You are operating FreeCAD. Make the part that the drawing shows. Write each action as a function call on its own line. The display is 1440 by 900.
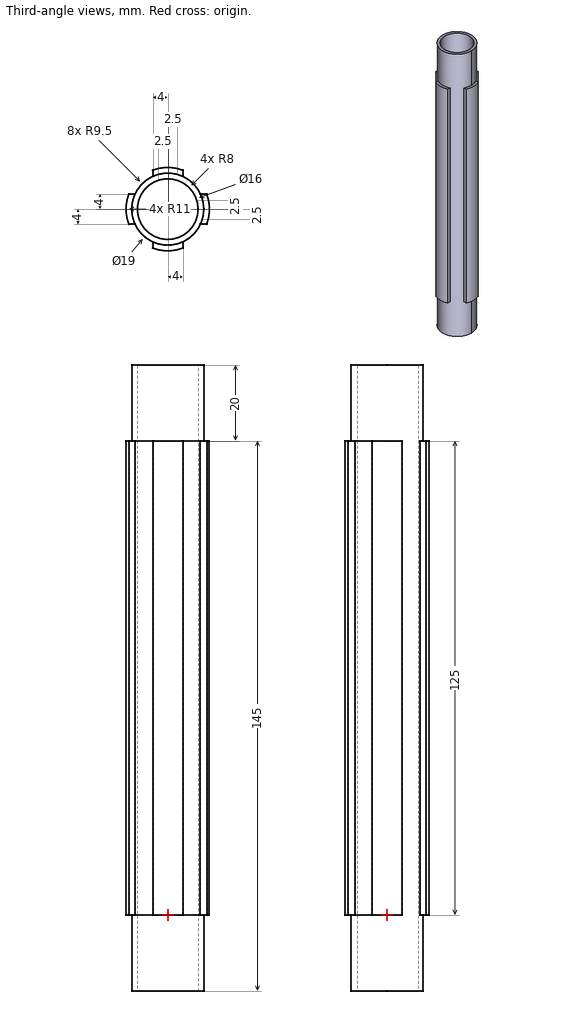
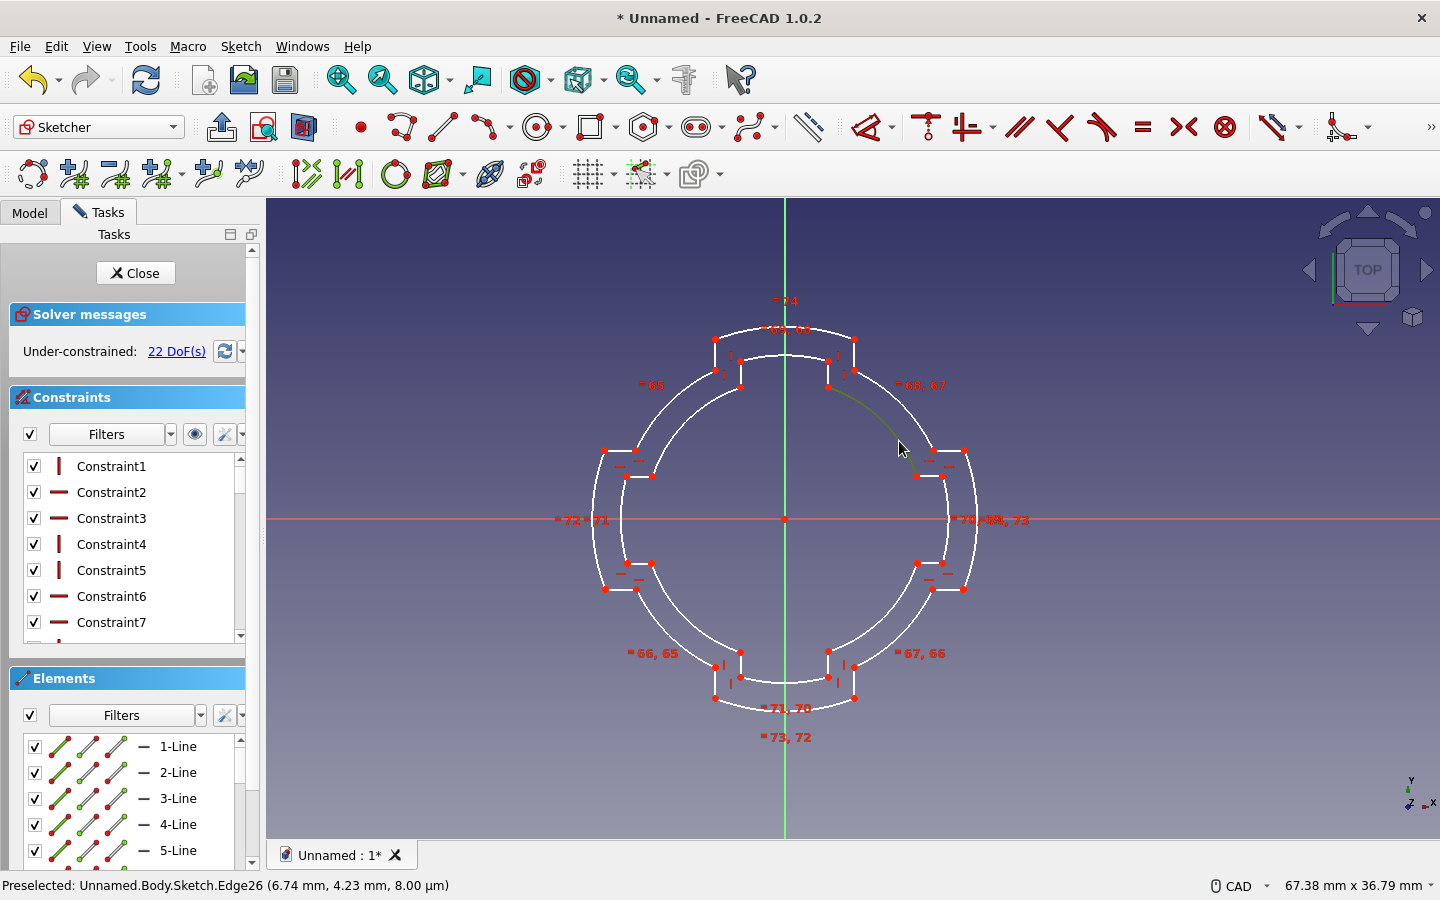
click(863, 635)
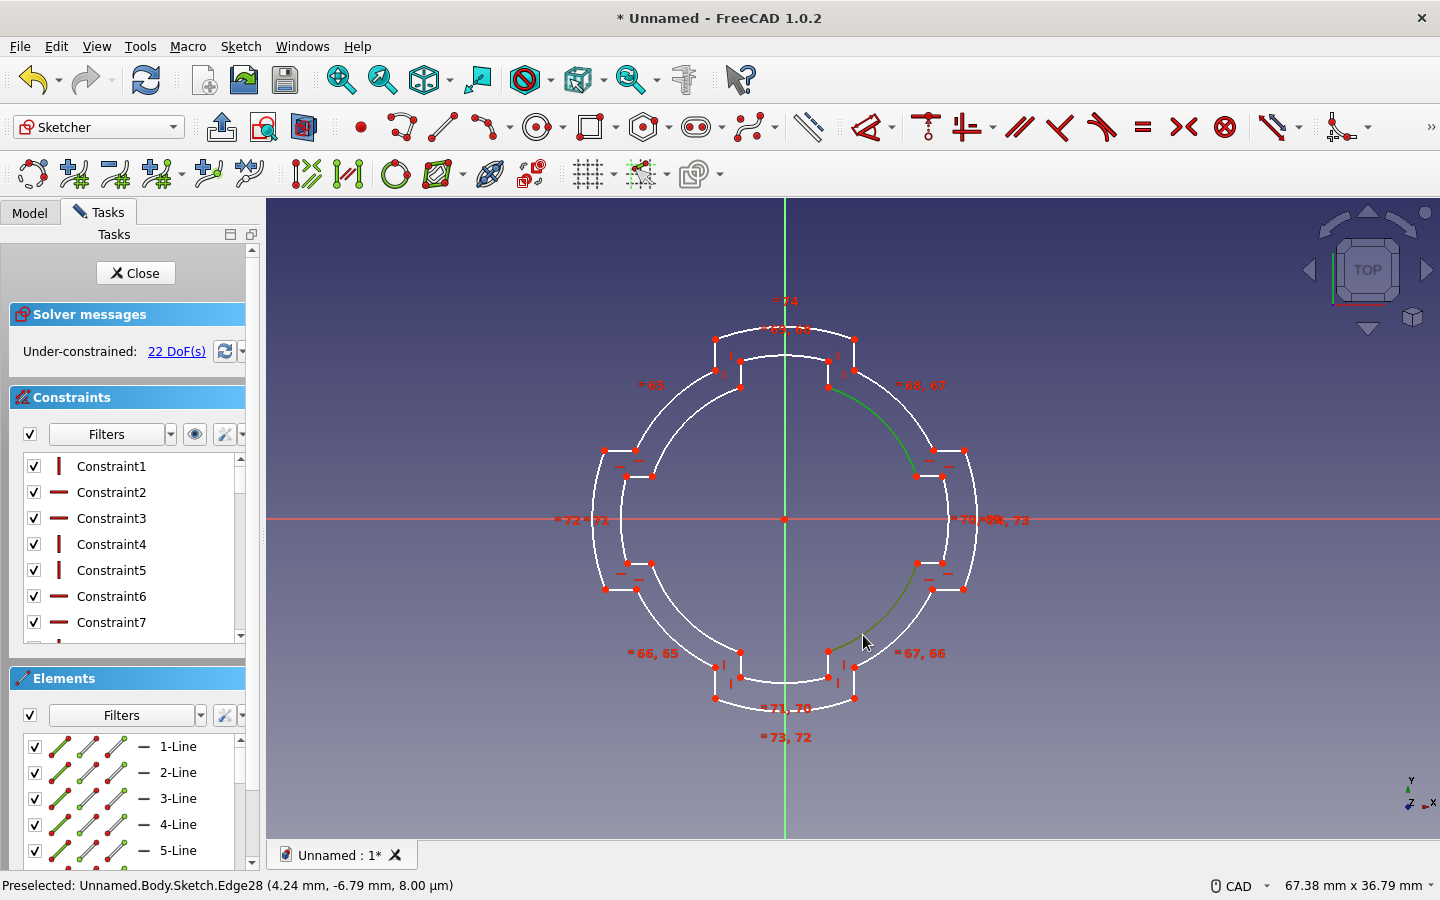
click(669, 599)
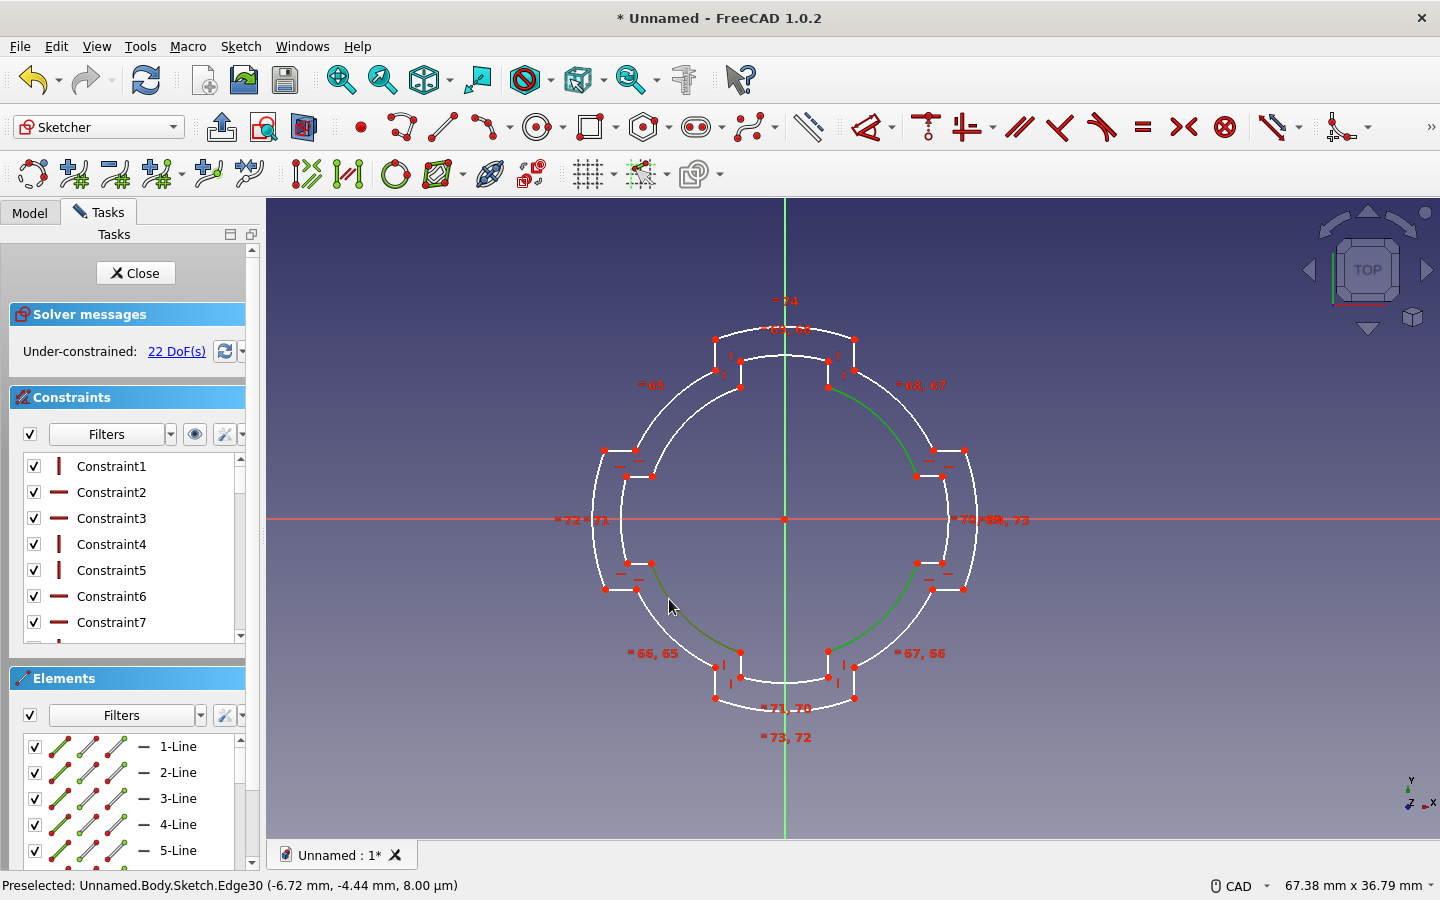
click(706, 405)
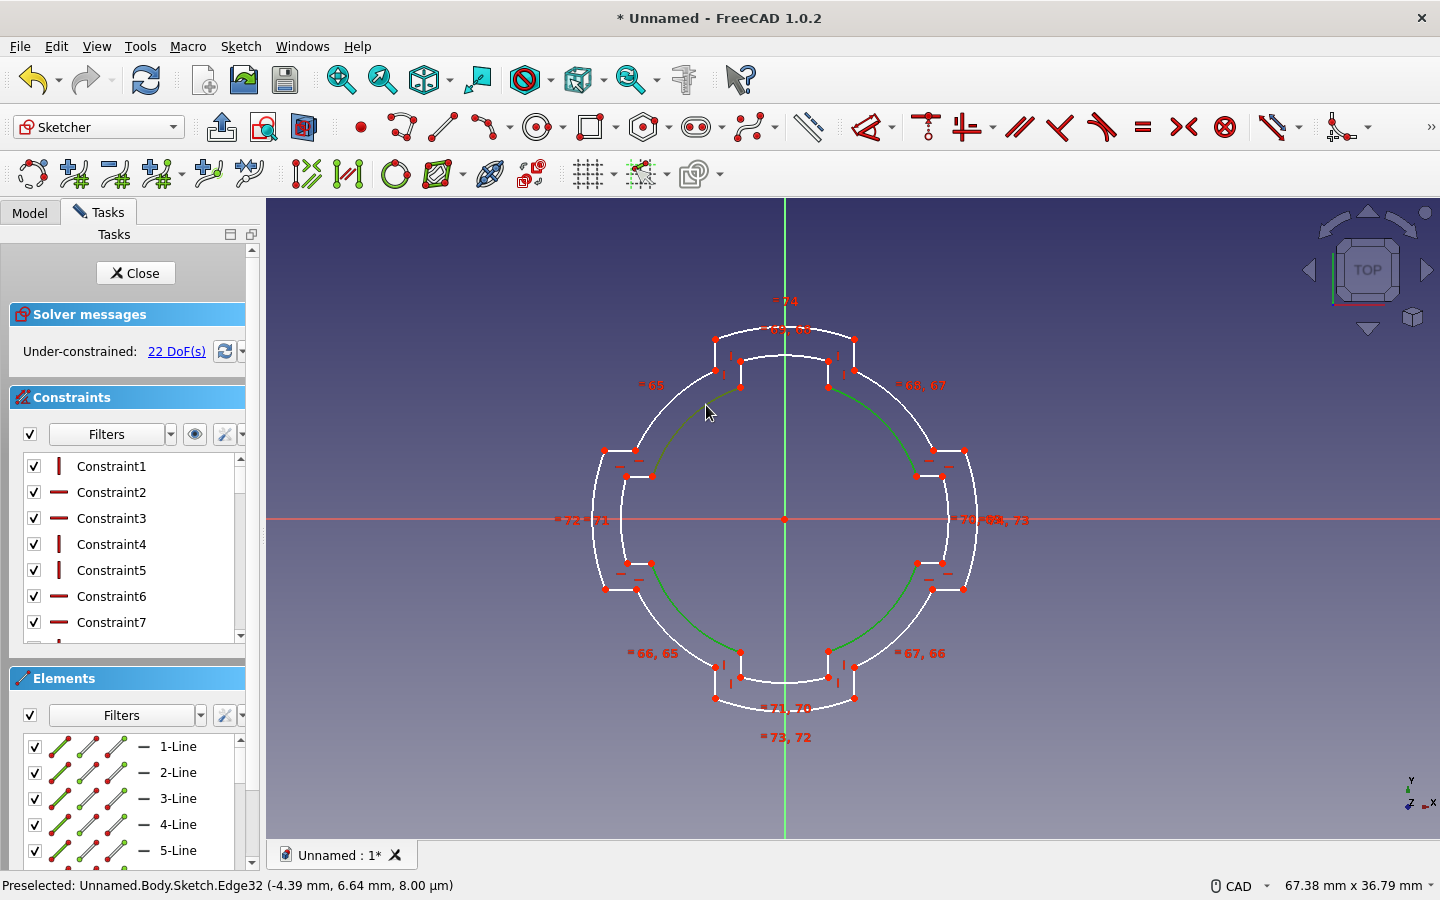
click(1143, 128)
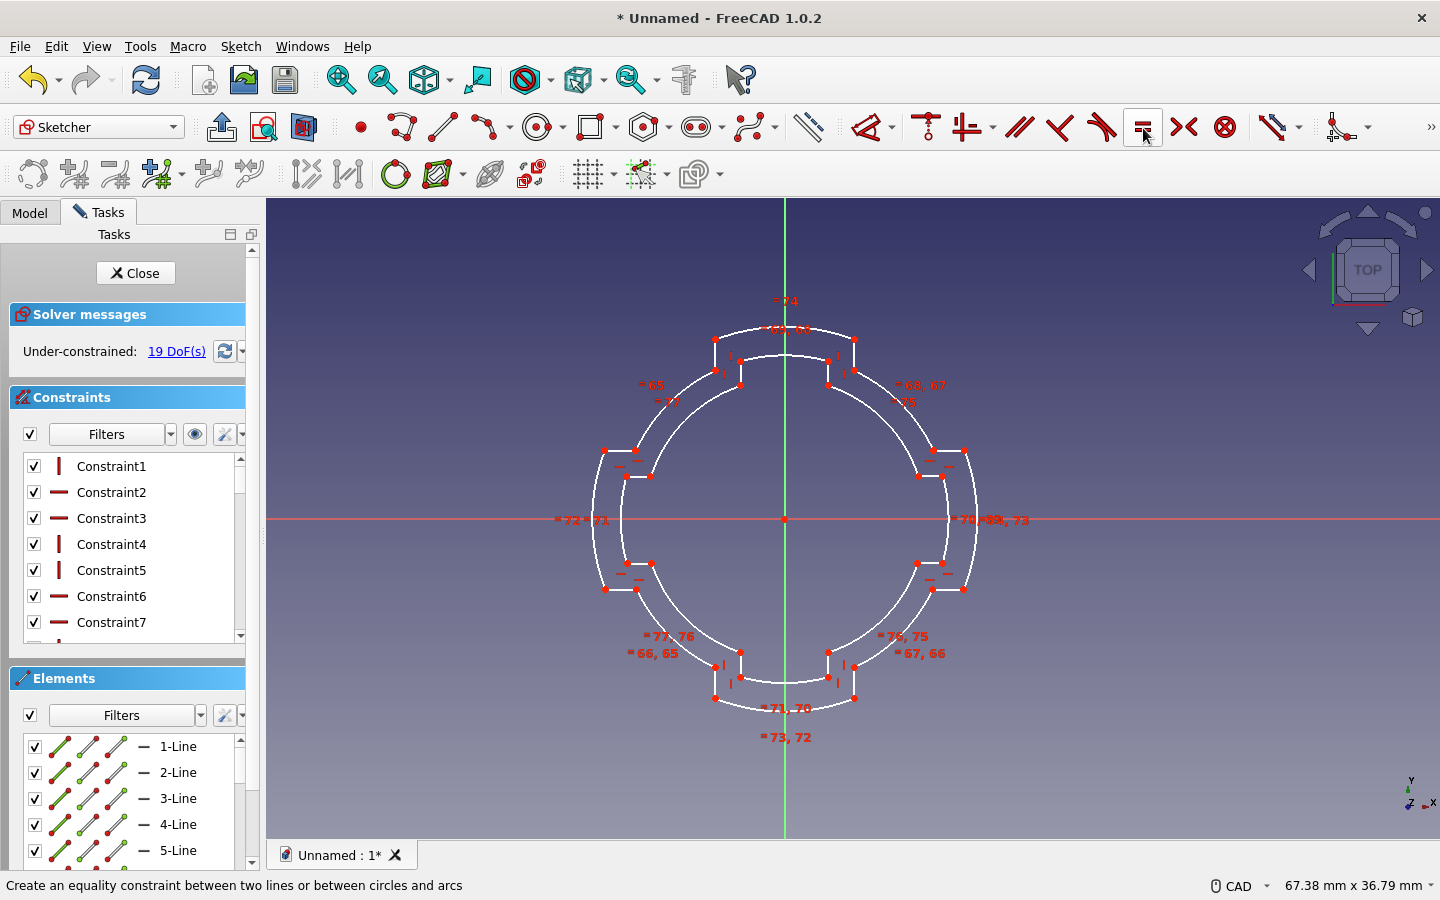
click(866, 128)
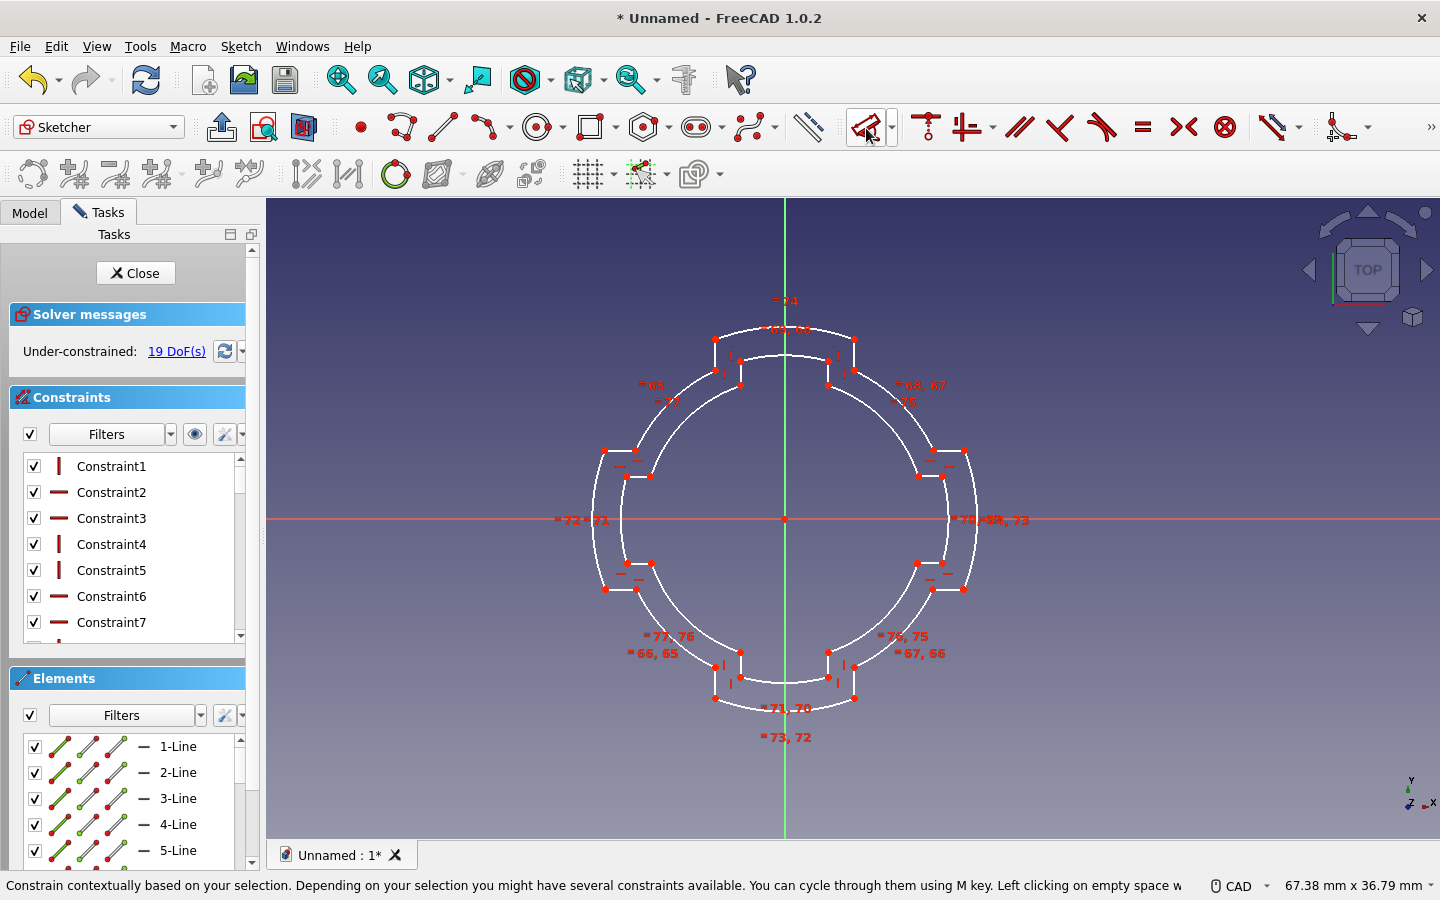
click(686, 389)
click(667, 363)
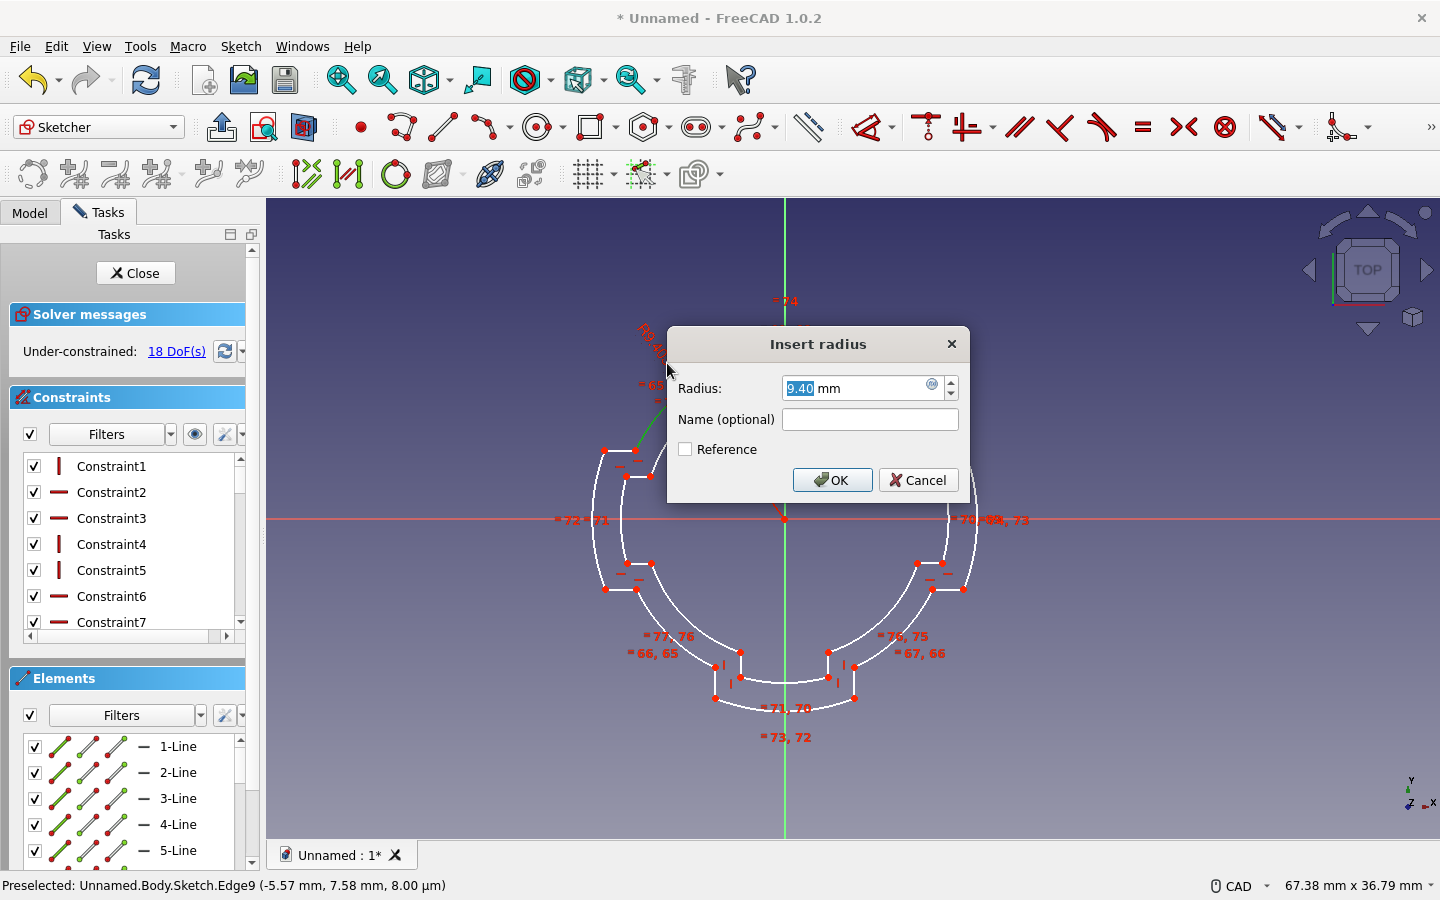
text(9.5)
key(Return)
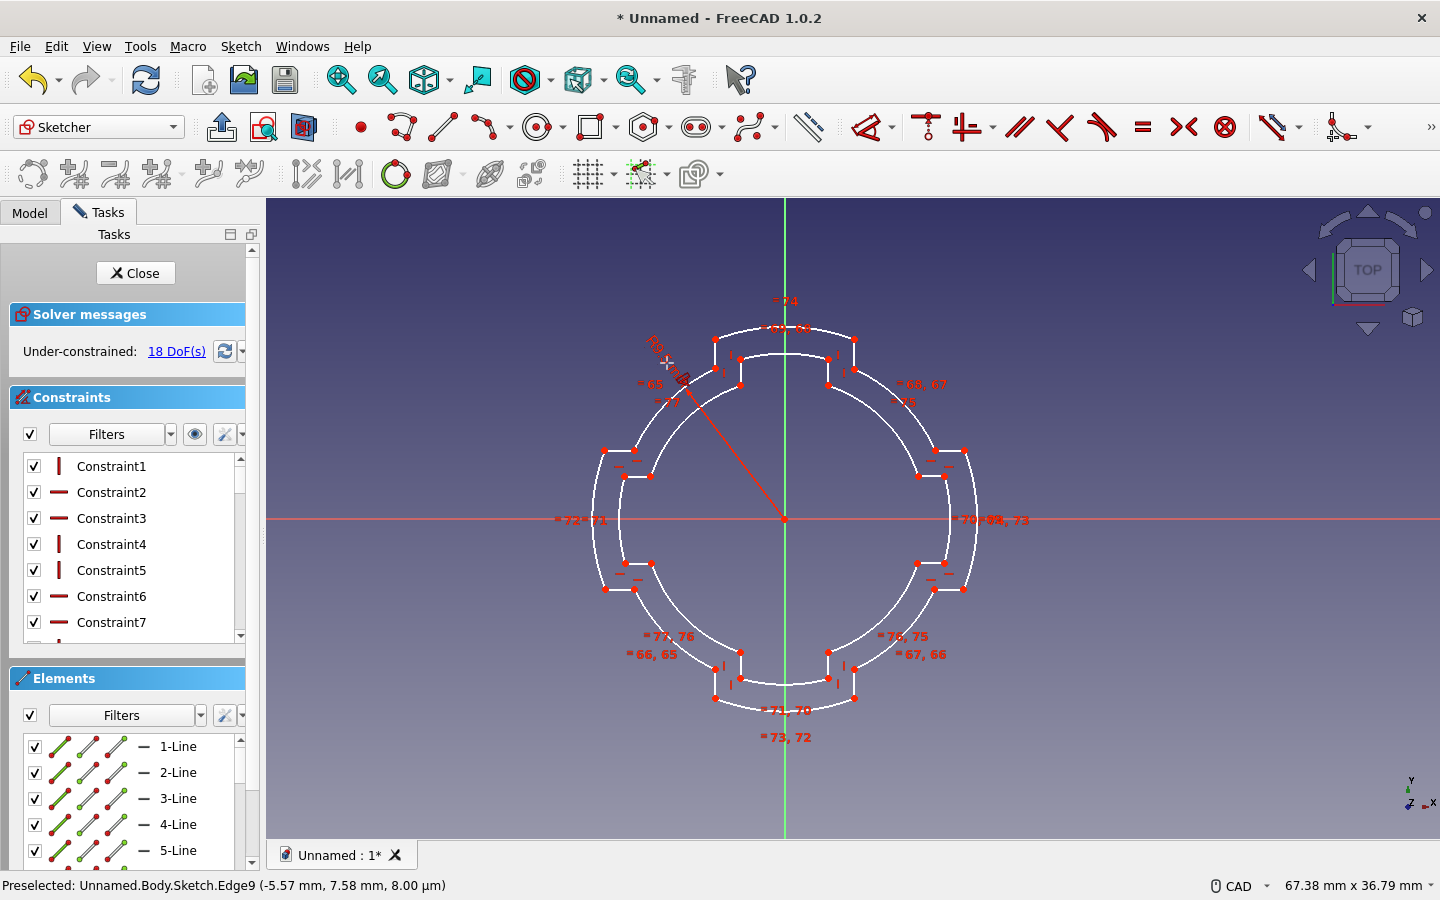
click(594, 492)
click(562, 487)